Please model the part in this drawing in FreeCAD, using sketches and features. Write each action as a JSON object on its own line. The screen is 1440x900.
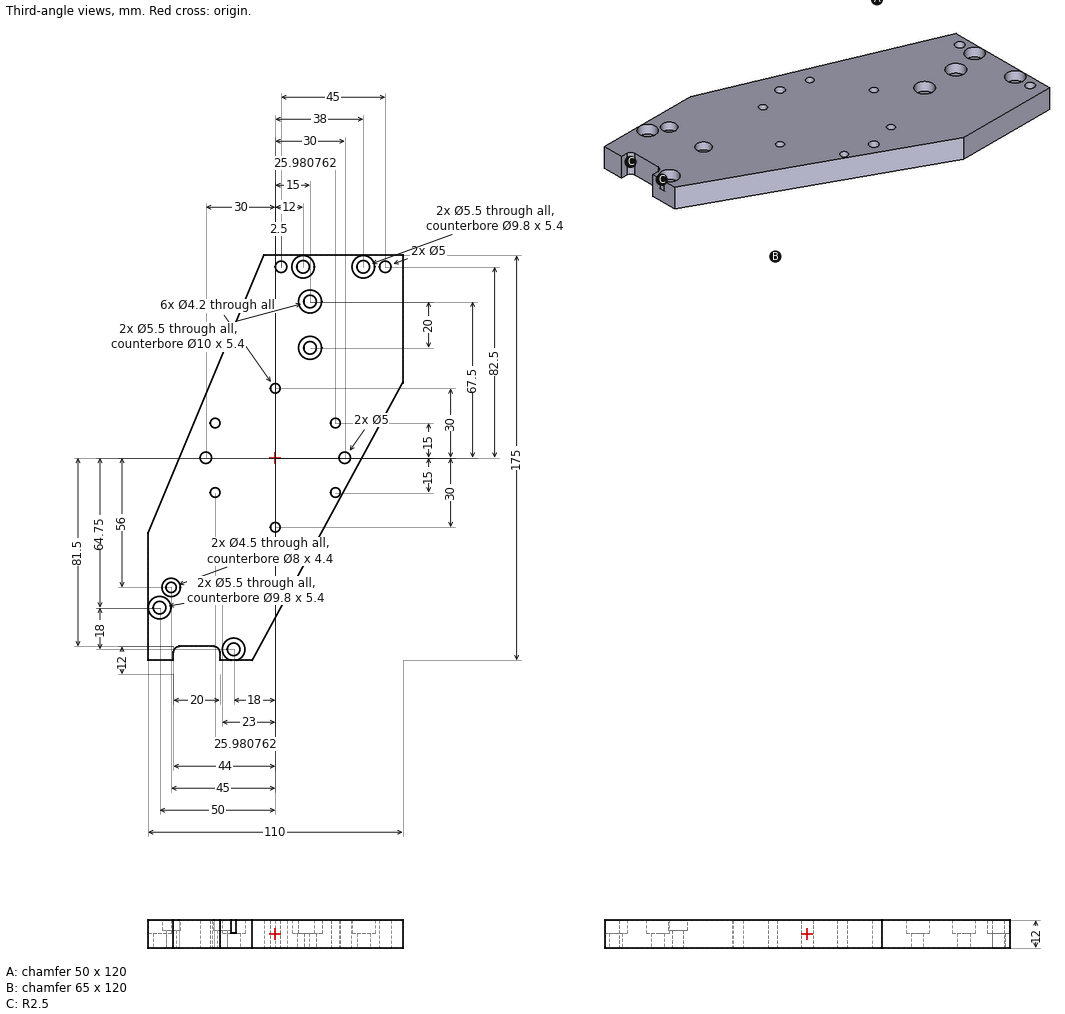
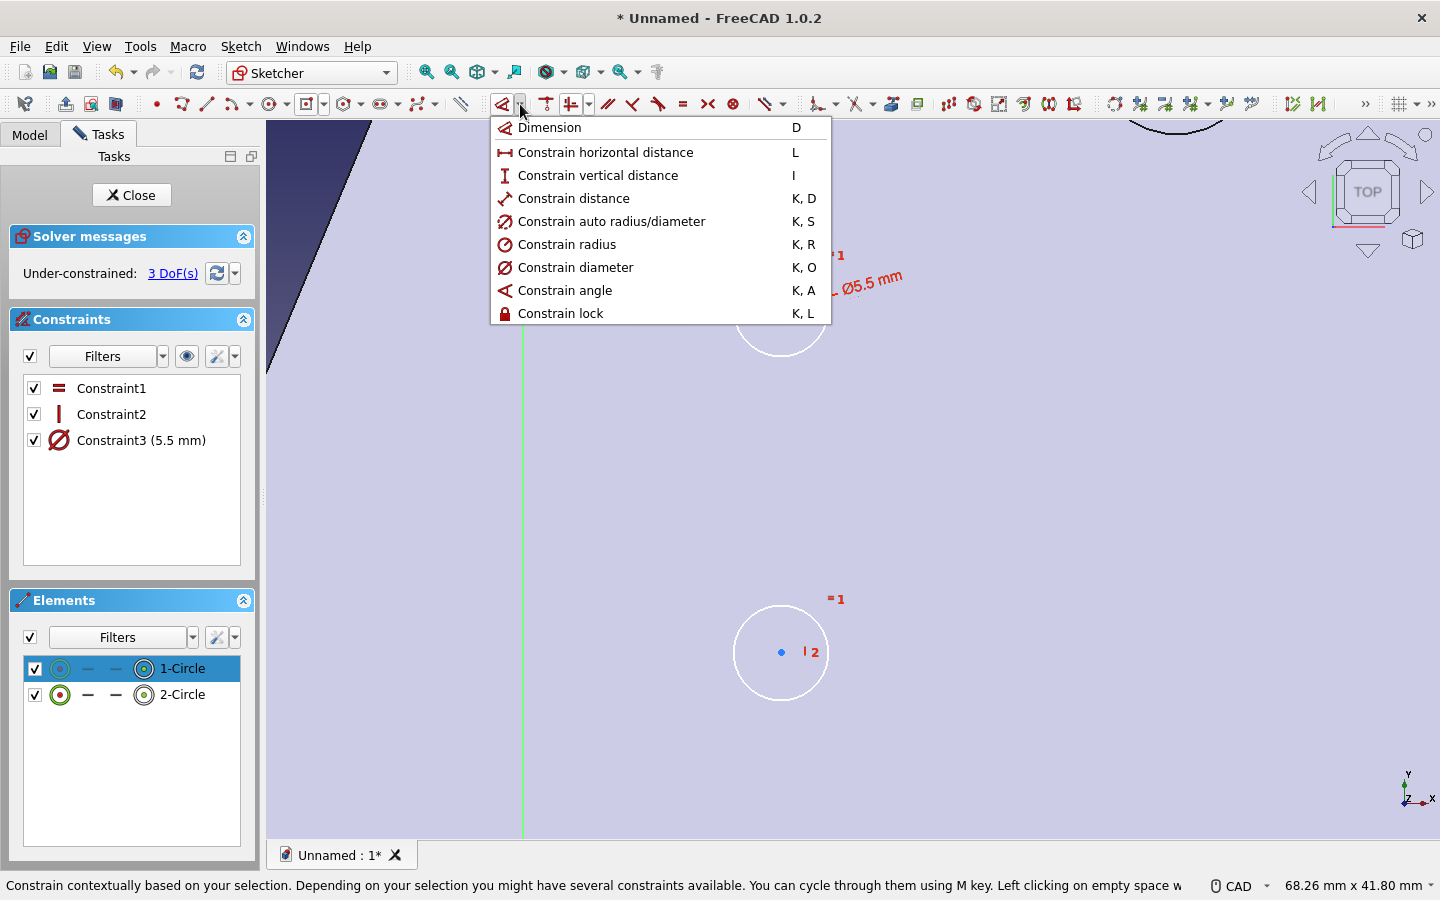
{"action": "left_click", "coordinate": [661, 152]}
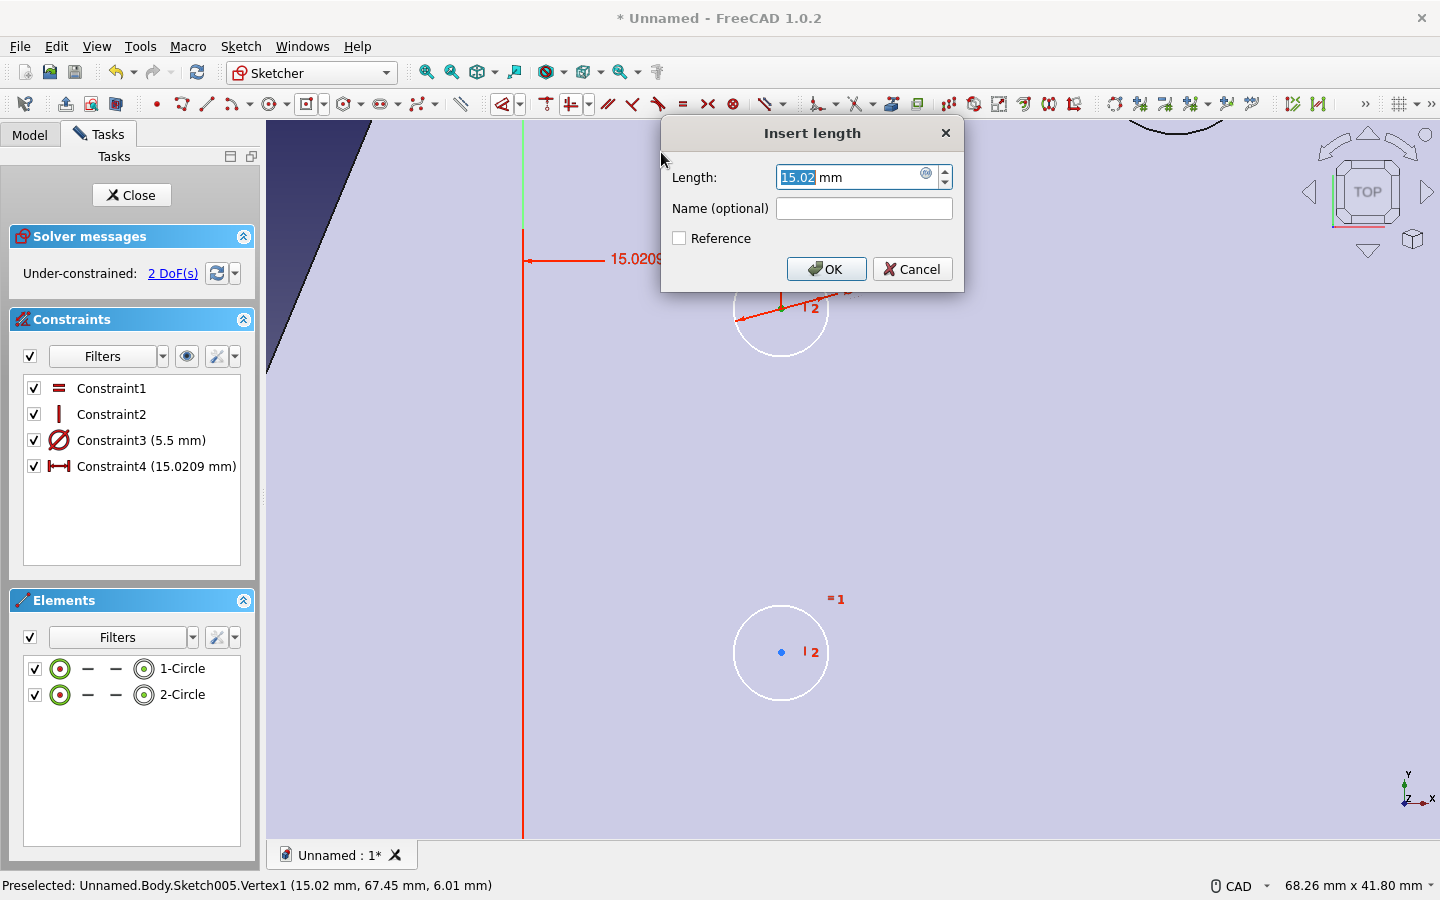
{"action": "type", "text": "15"}
{"action": "key", "text": "Return"}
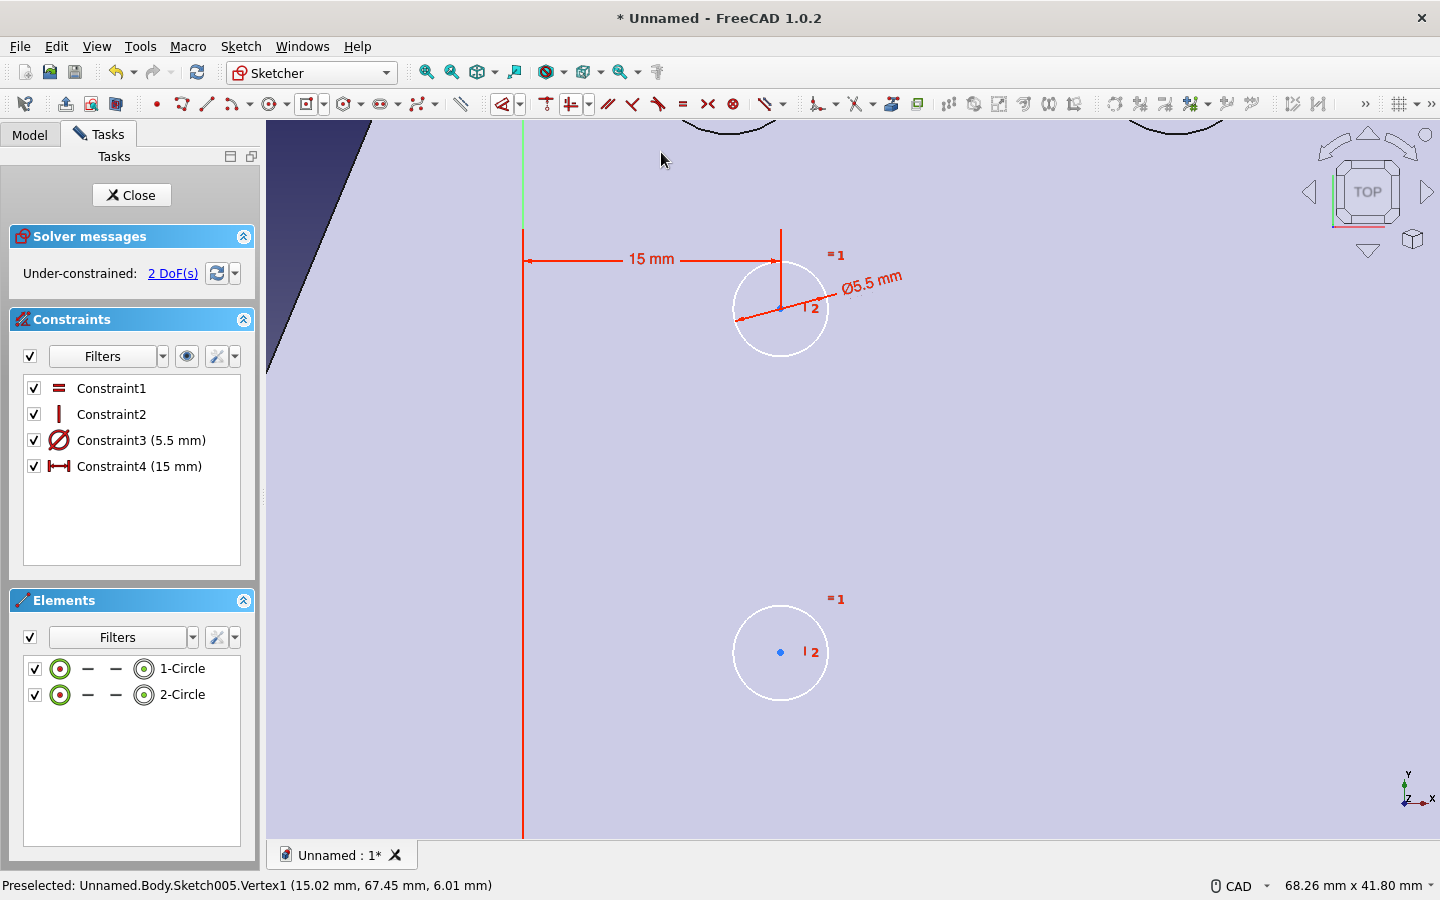
{"action": "left_click", "coordinate": [781, 309]}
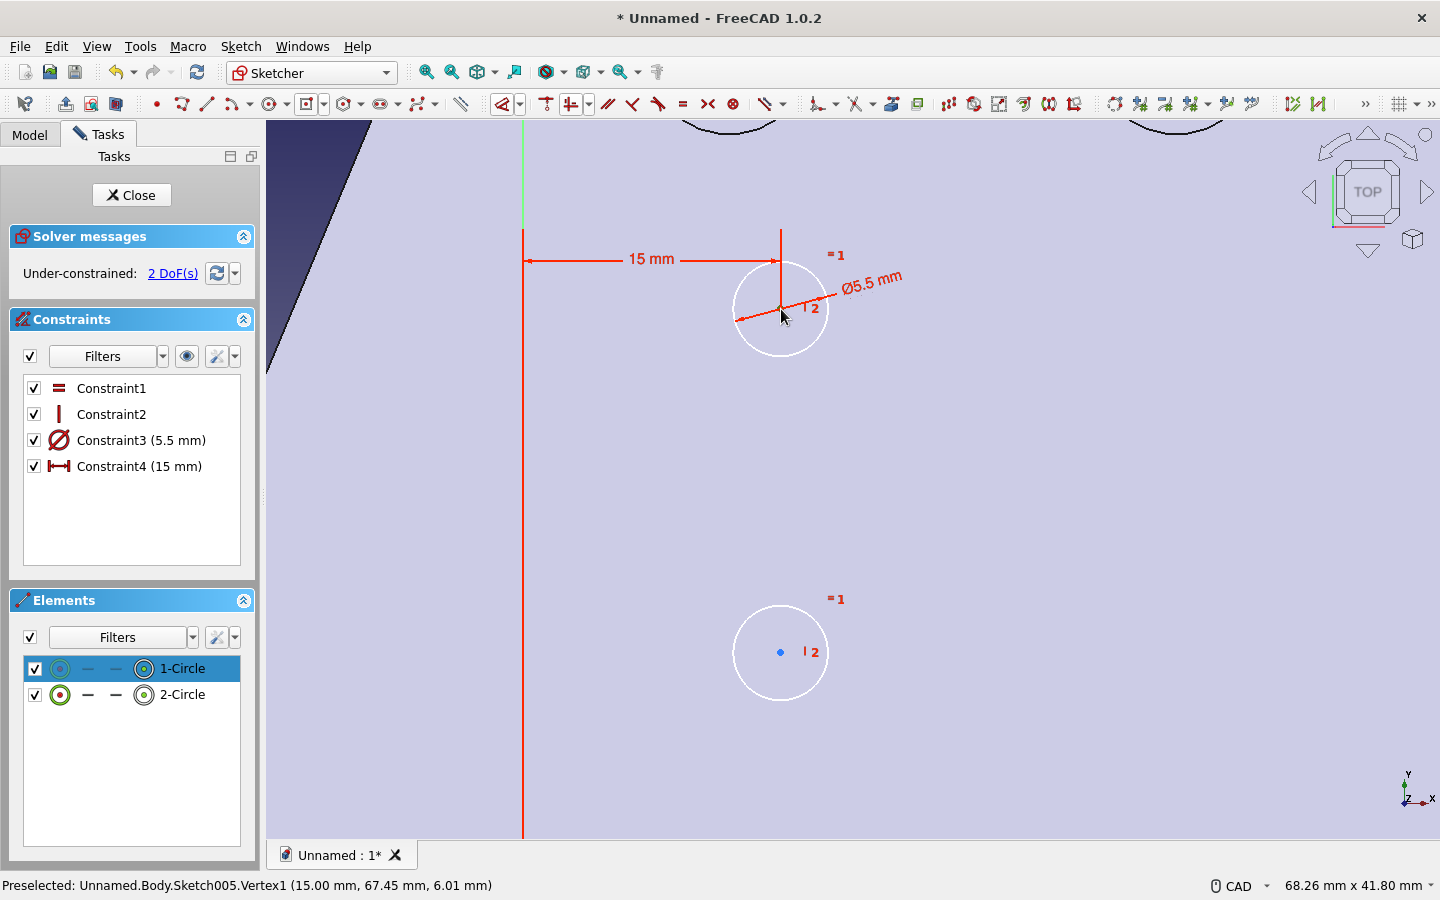
{"action": "left_click", "coordinate": [781, 653]}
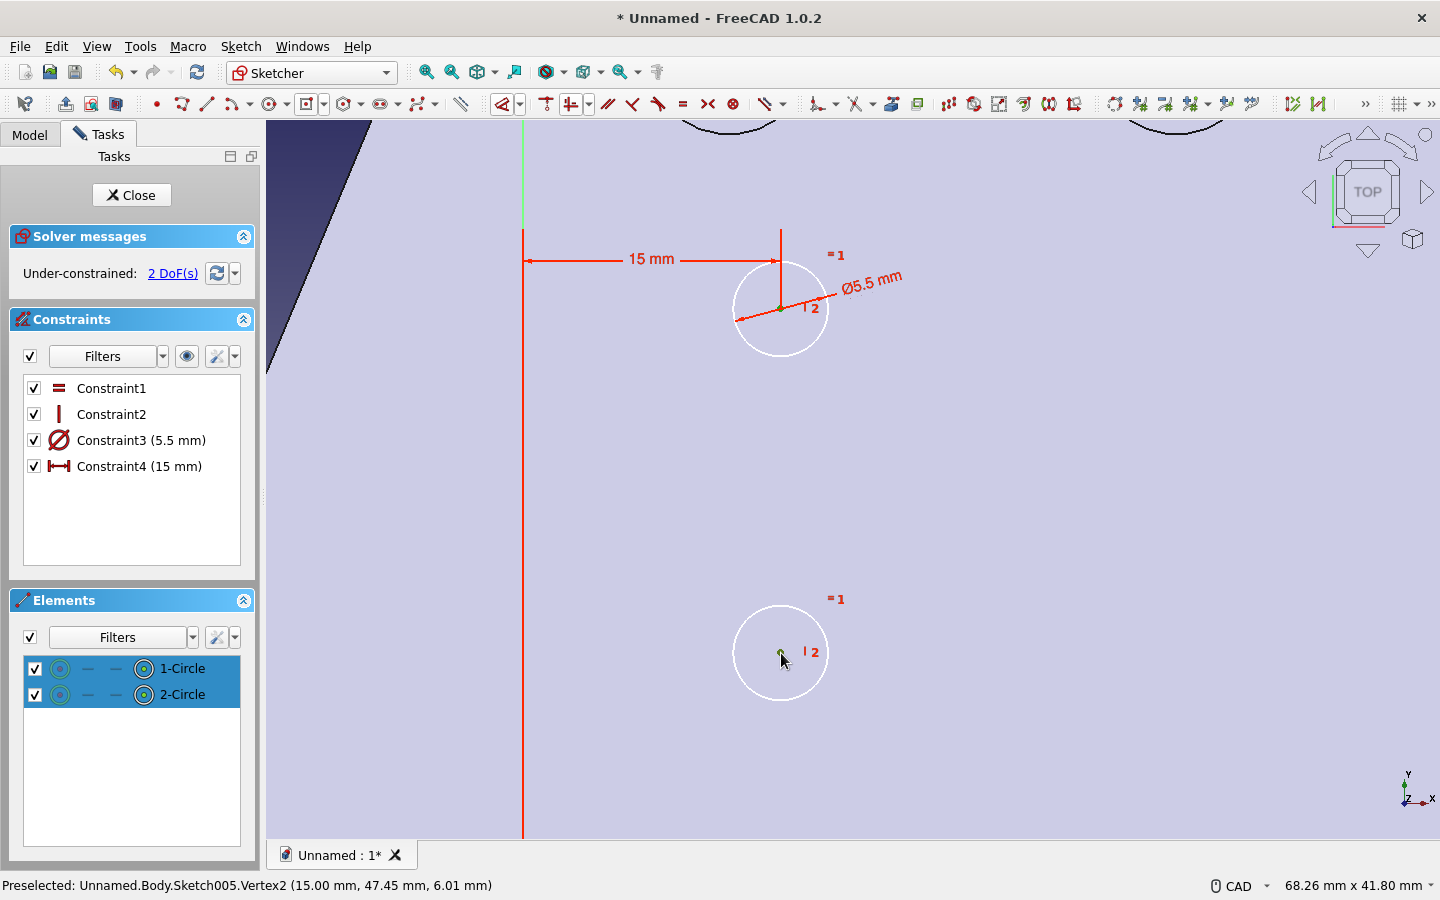
{"action": "key", "text": "i"}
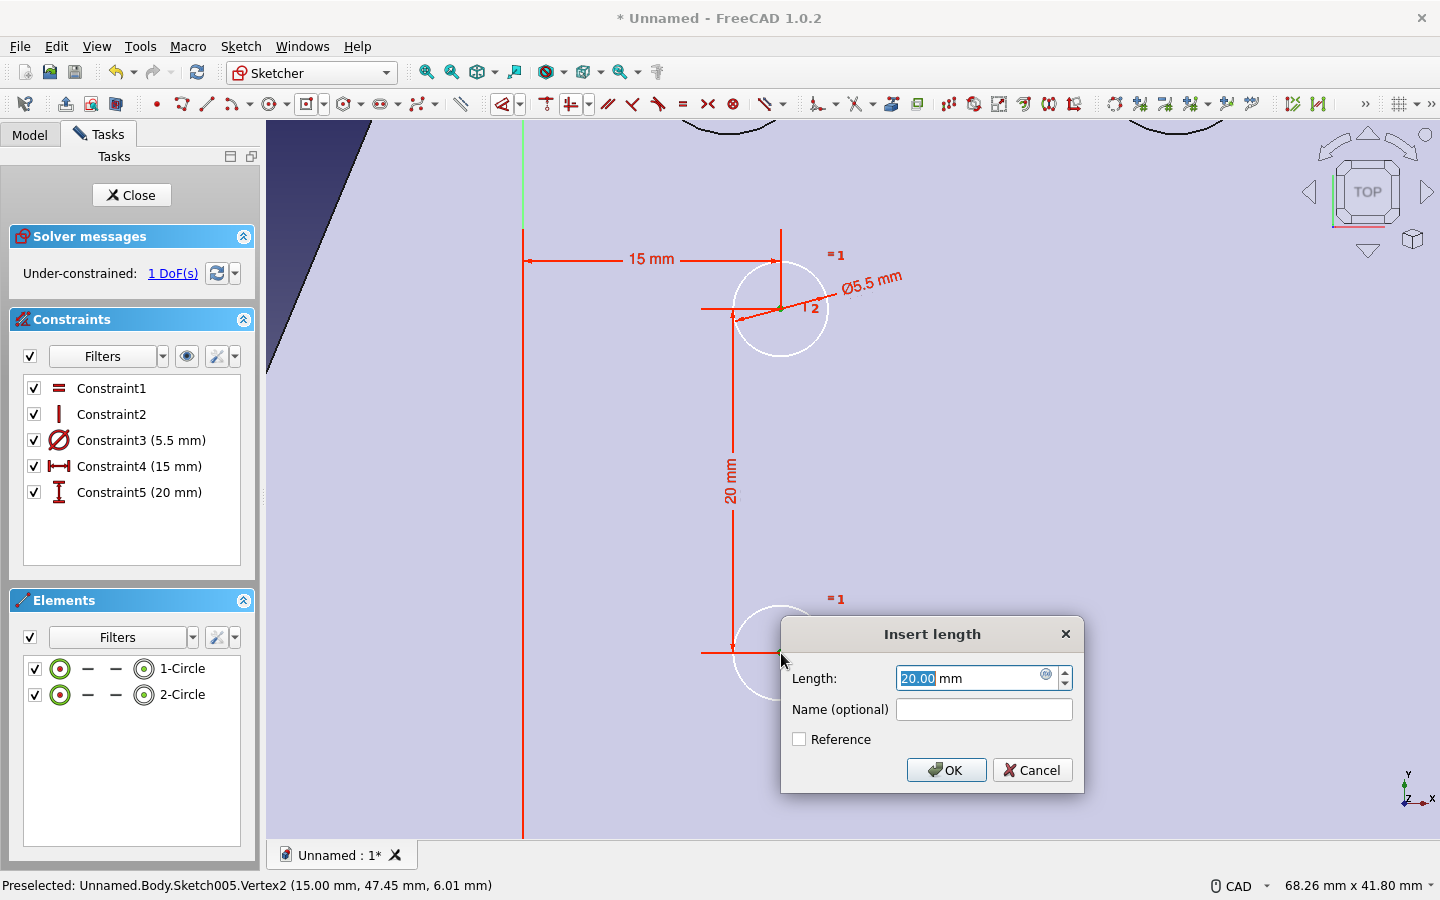
{"action": "type", "text": "20"}
{"action": "key", "text": "Return"}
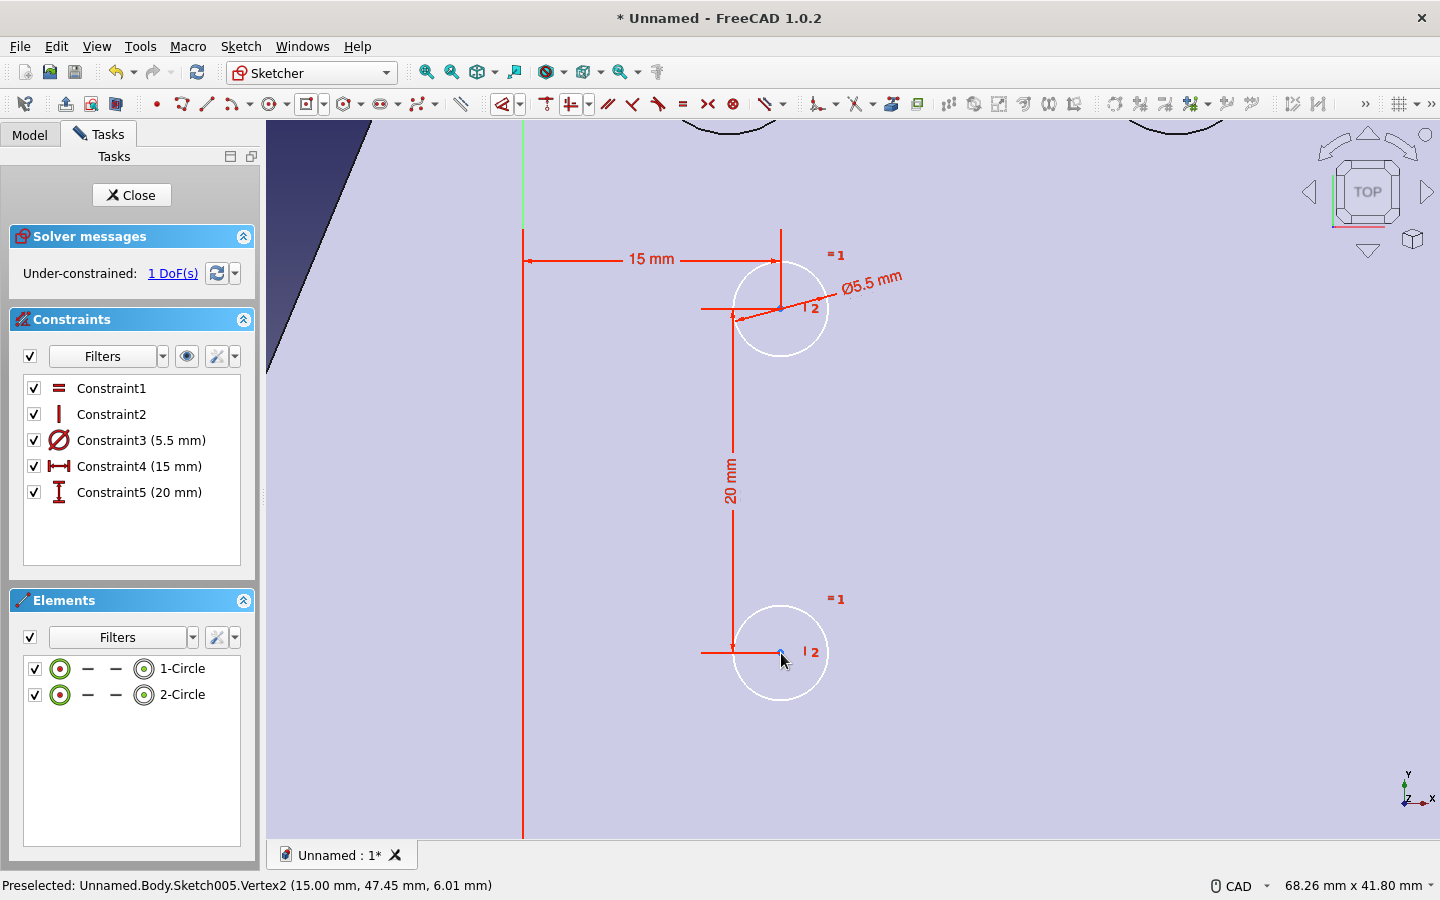
{"action": "left_click", "coordinate": [781, 309]}